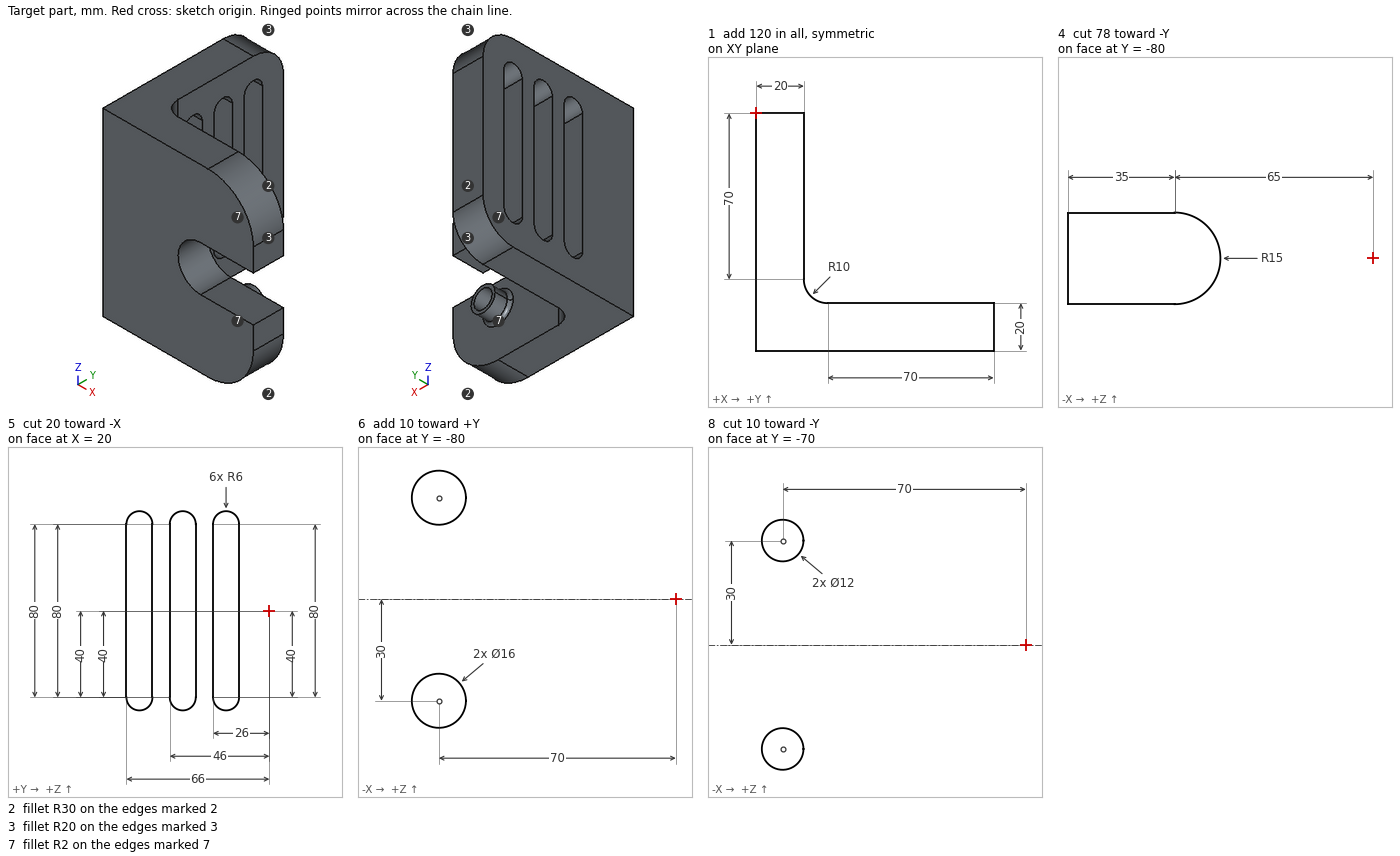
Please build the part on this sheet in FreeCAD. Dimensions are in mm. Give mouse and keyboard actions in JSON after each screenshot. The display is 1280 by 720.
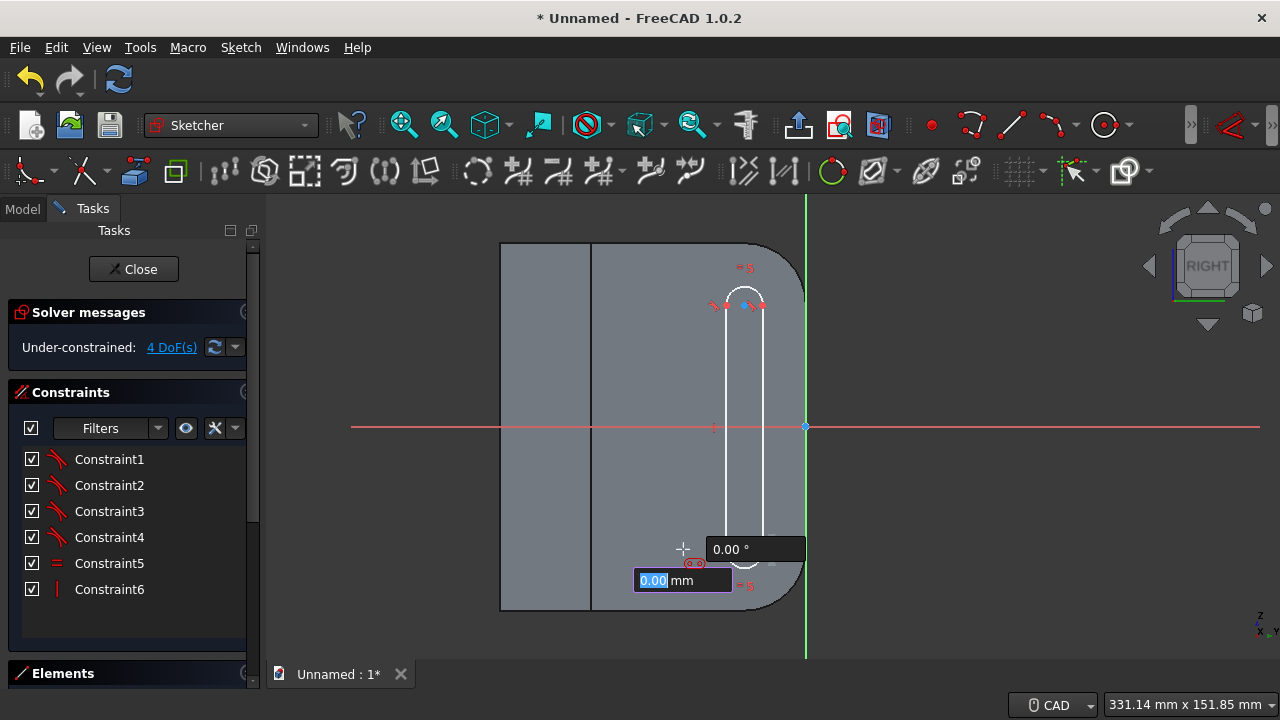
{"action": "left_click", "coordinate": [683, 304]}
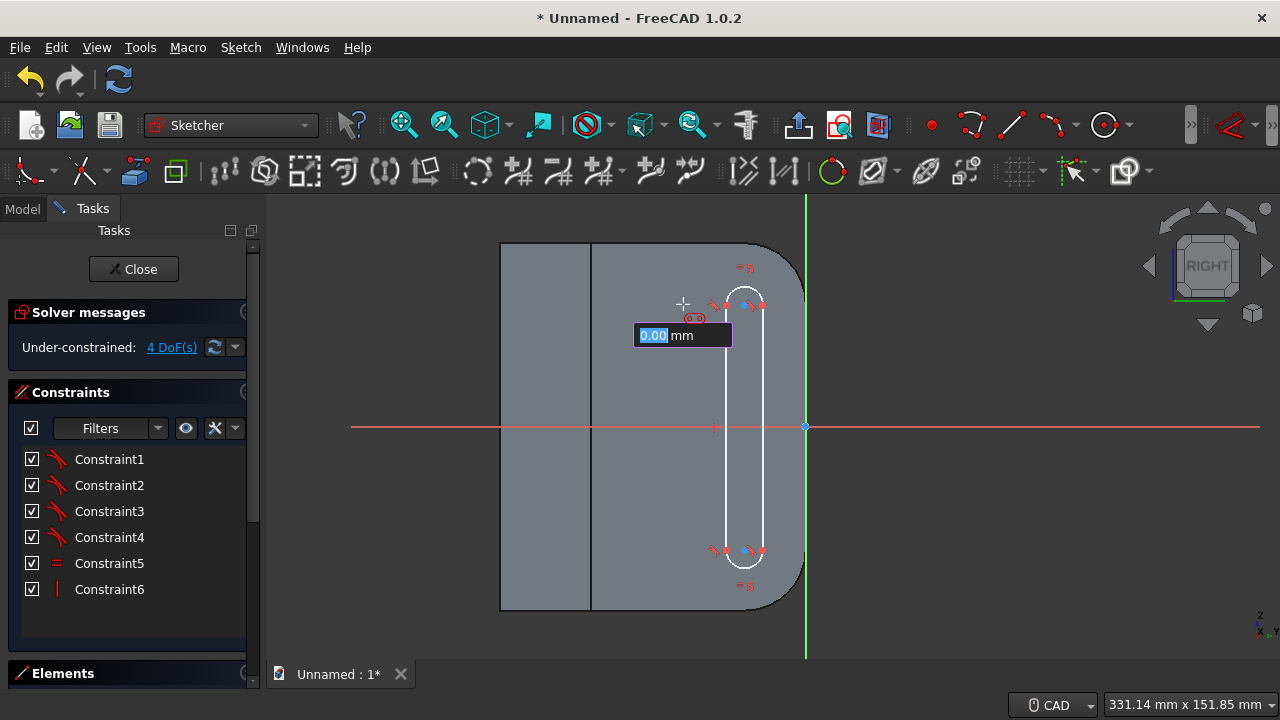
{"action": "left_click", "coordinate": [665, 390]}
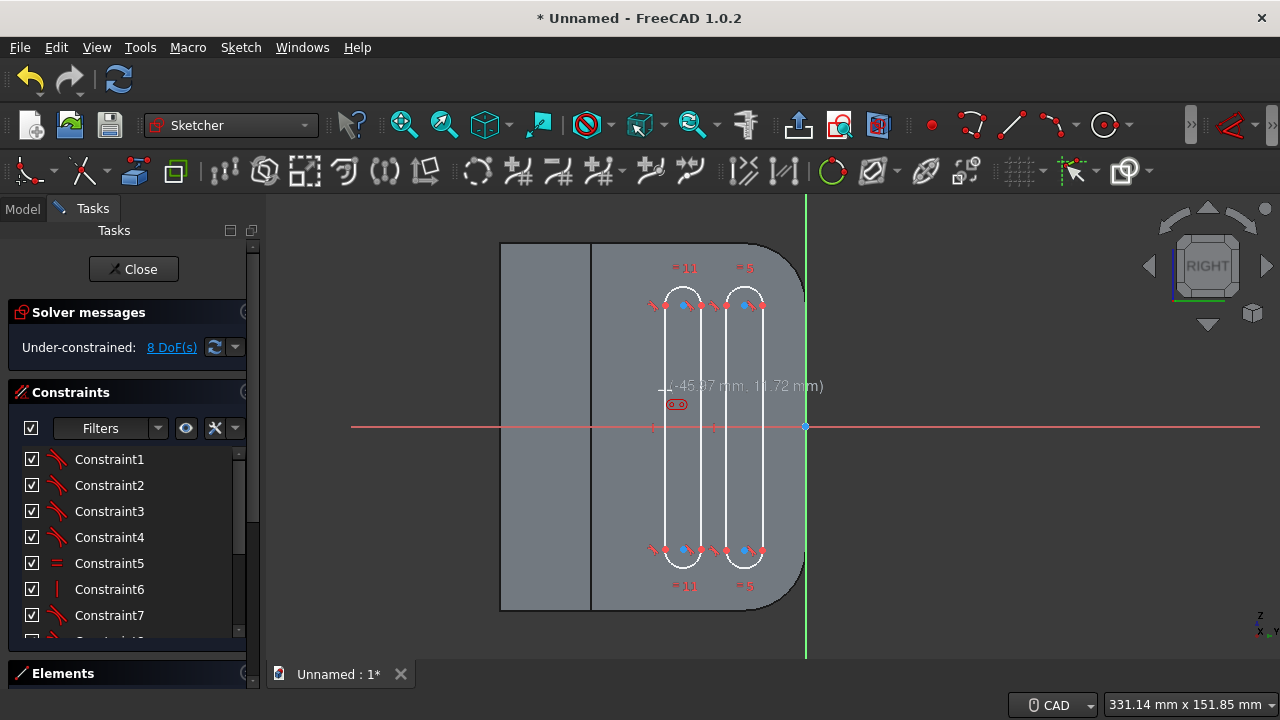
{"action": "scroll", "coordinate": [622, 549], "scroll_direction": "up", "scroll_amount": 2}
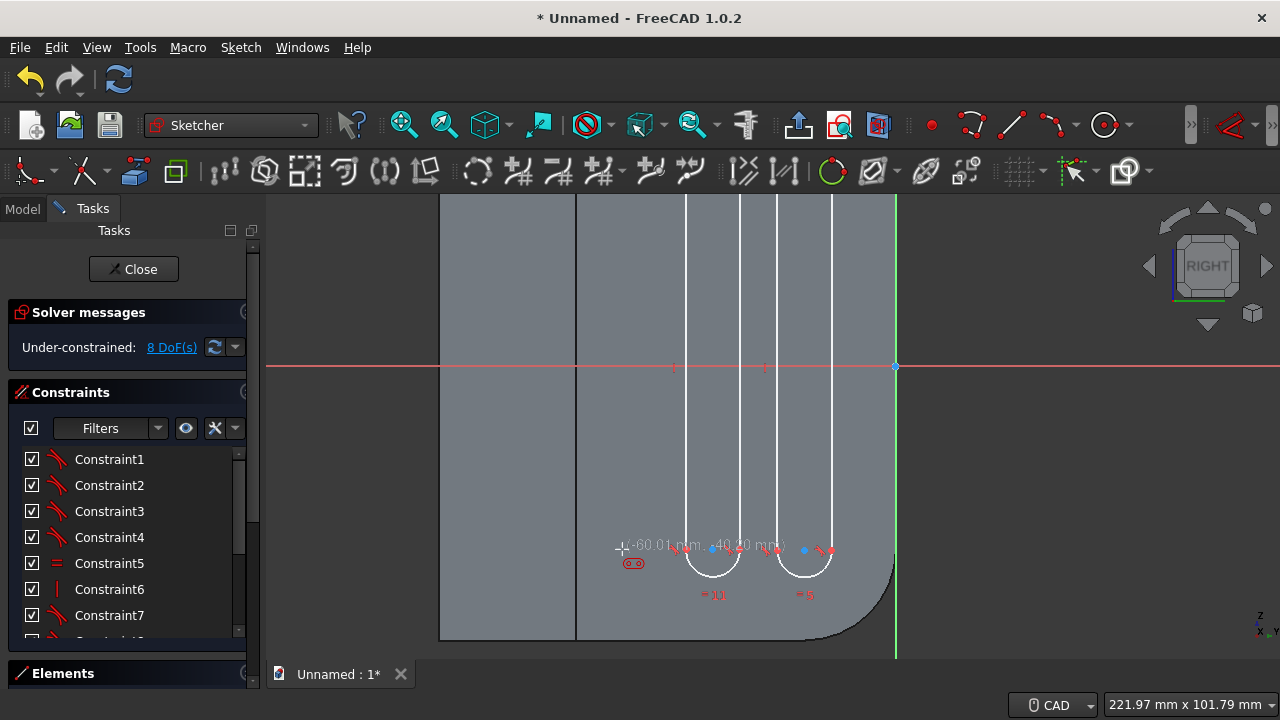
{"action": "left_click", "coordinate": [622, 549]}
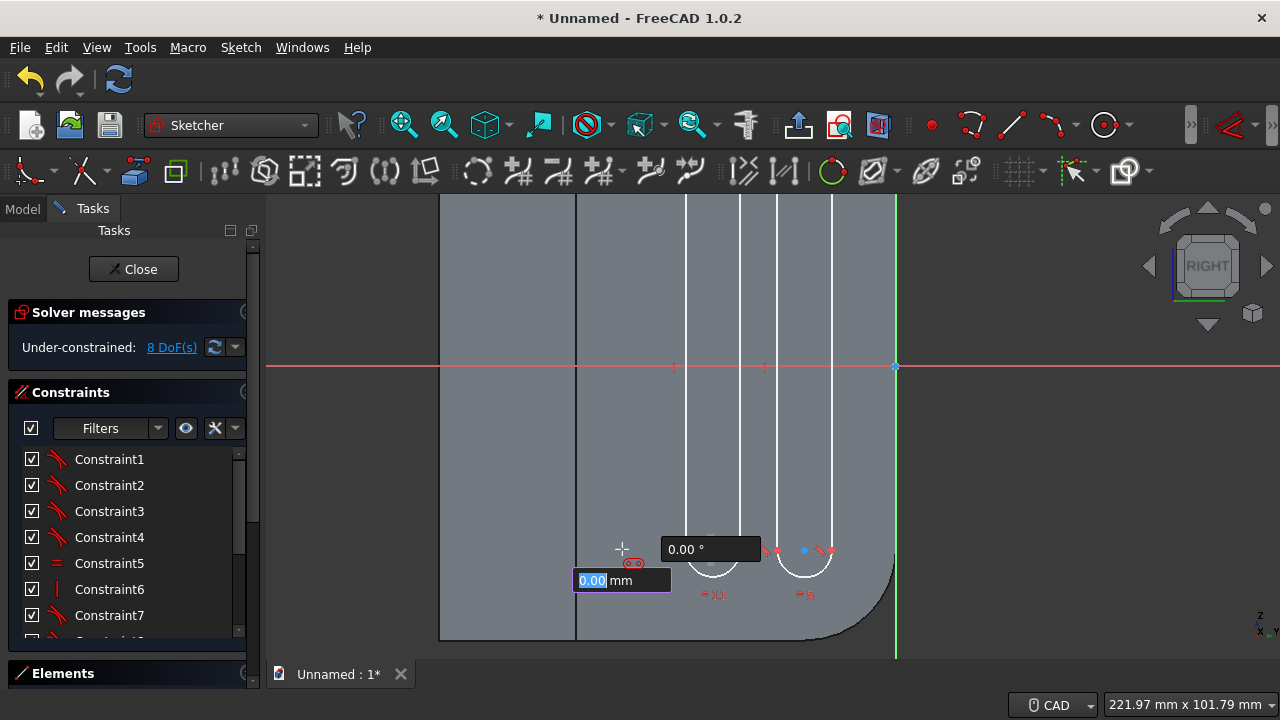
{"action": "scroll", "coordinate": [622, 549], "scroll_direction": "down", "scroll_amount": 2}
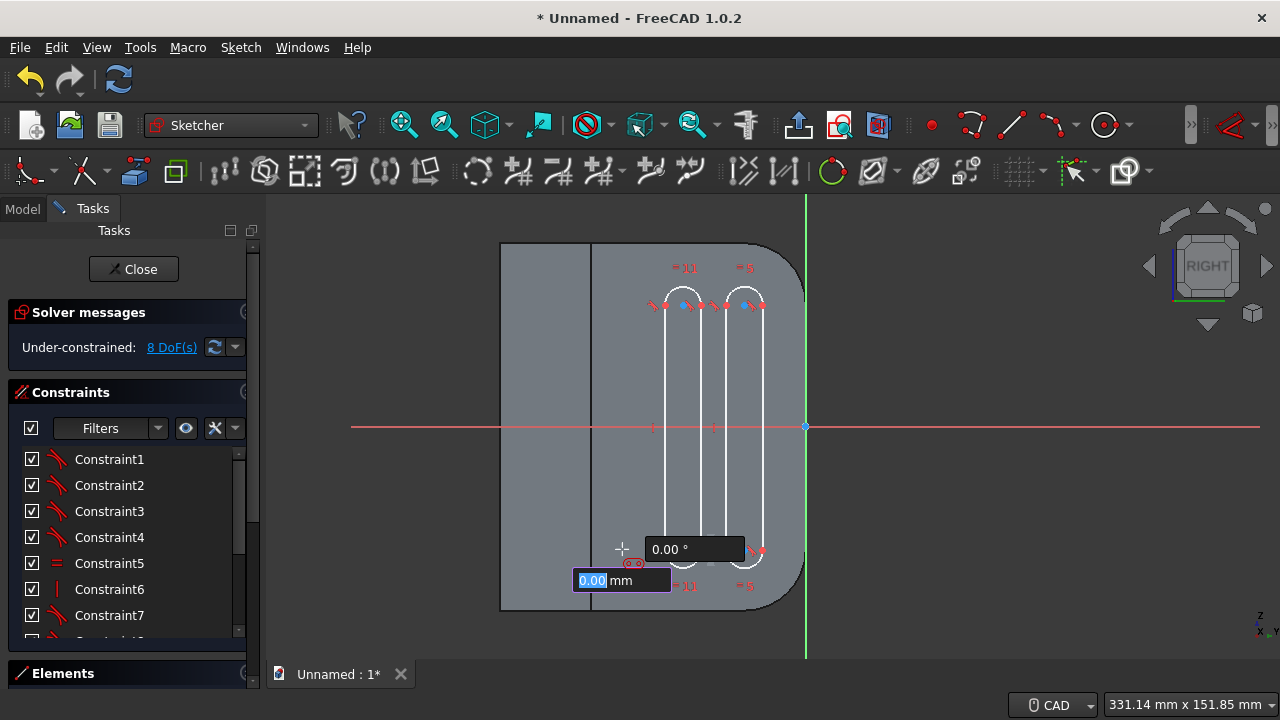
{"action": "left_click", "coordinate": [622, 304]}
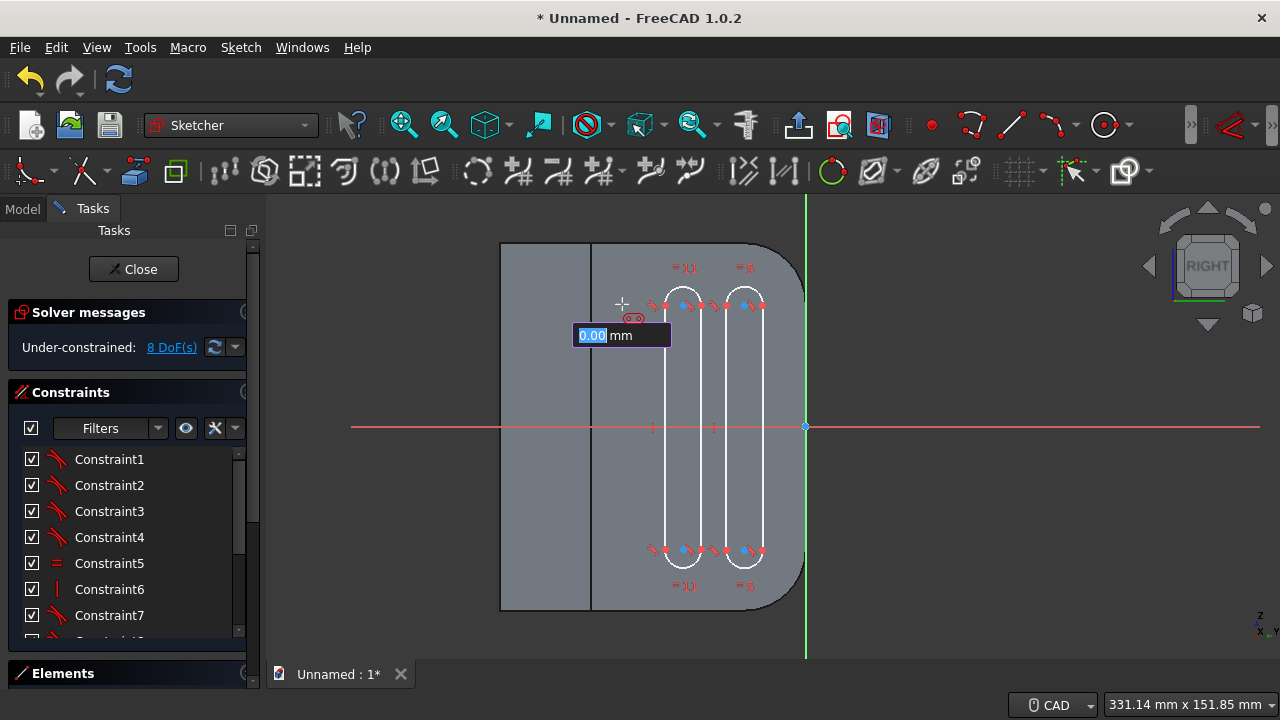
{"action": "left_click", "coordinate": [604, 390]}
{"action": "key", "text": "Escape"}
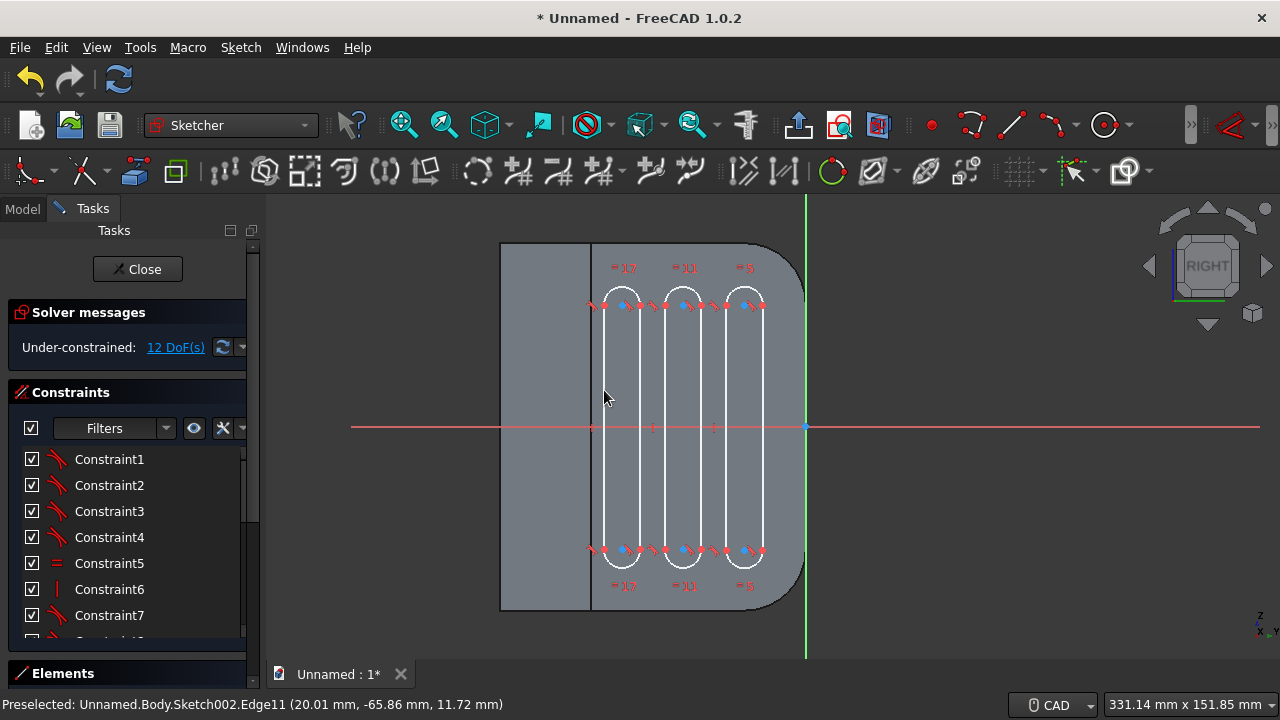
{"action": "left_click", "coordinate": [734, 565]}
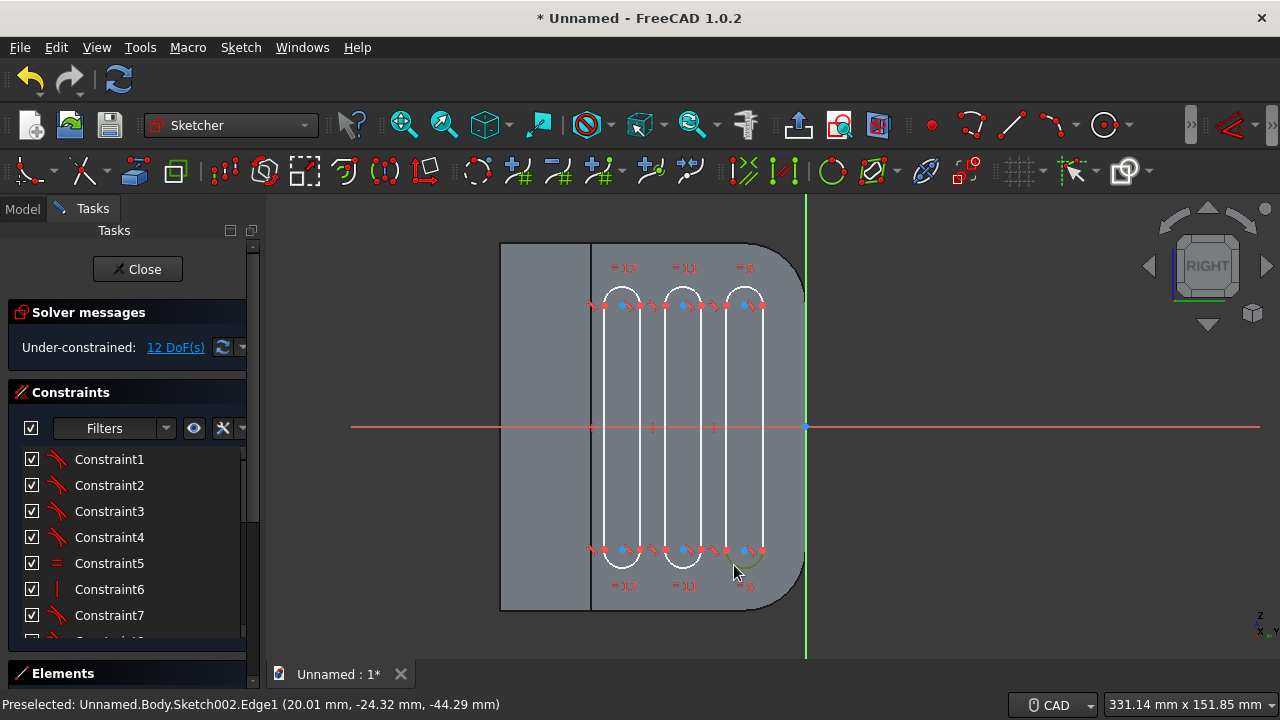
{"action": "left_click", "coordinate": [672, 564]}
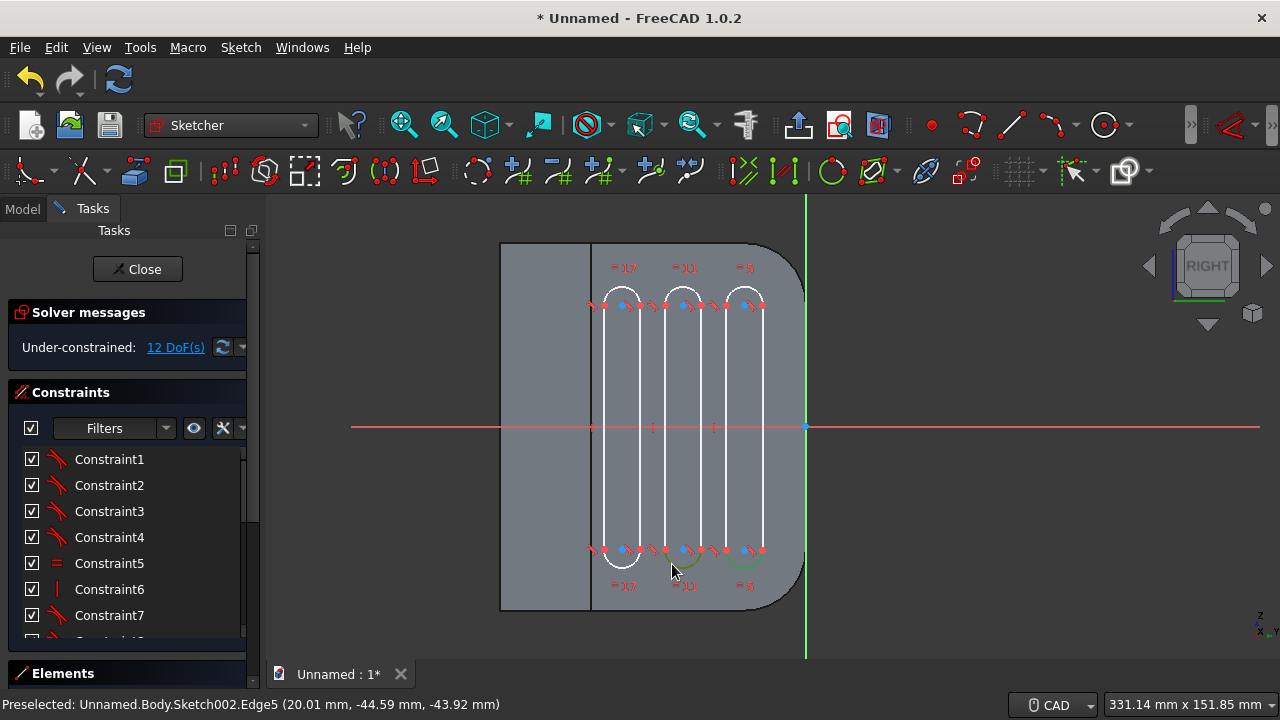
{"action": "left_click", "coordinate": [611, 564]}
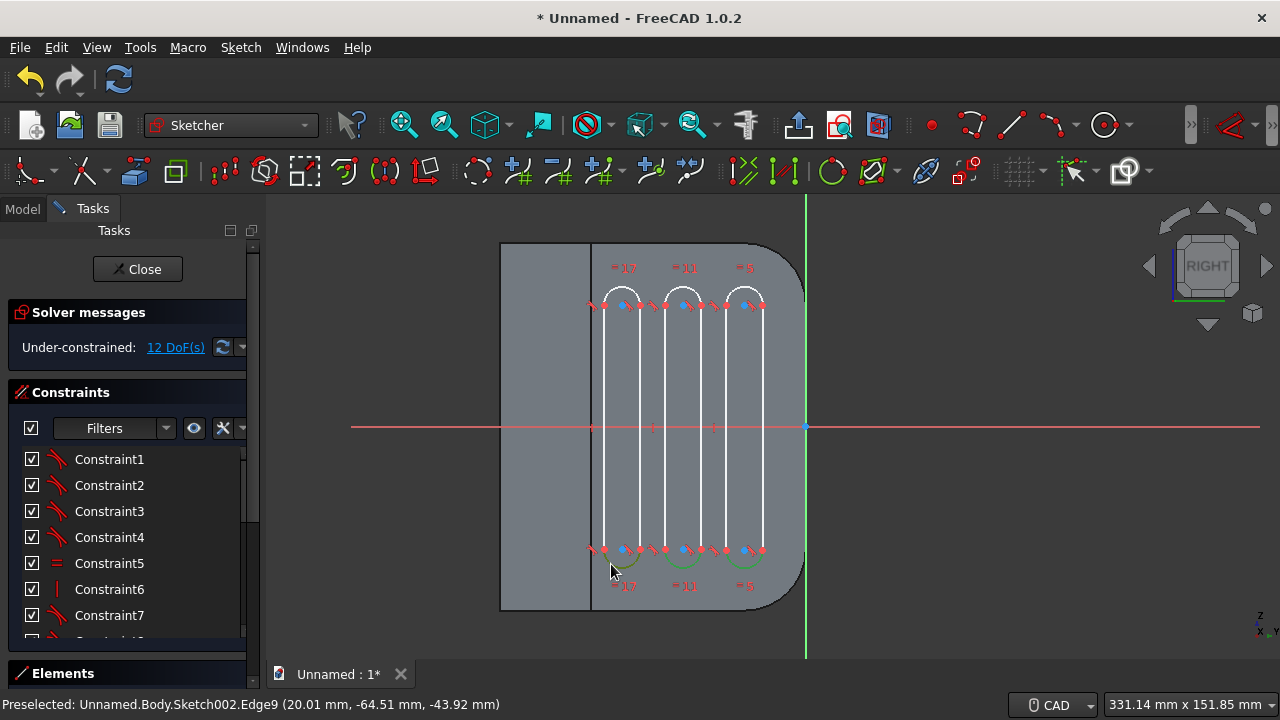
{"action": "key", "text": "e"}